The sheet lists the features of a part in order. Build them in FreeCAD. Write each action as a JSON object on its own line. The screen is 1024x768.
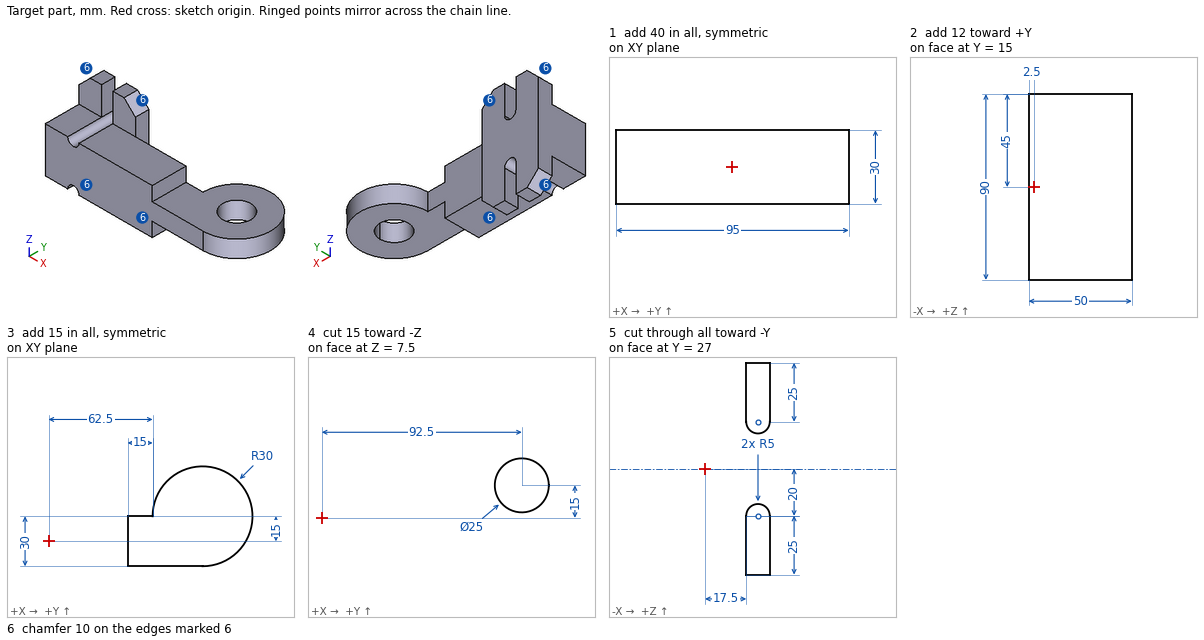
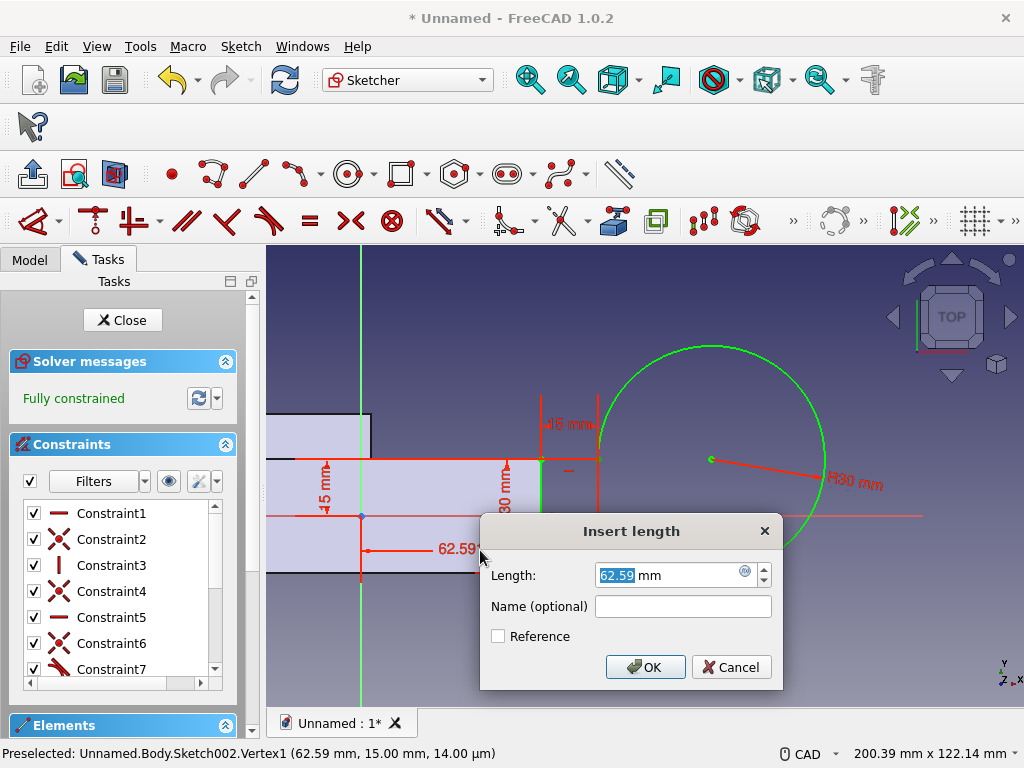
{"action": "type", "text": "62.5"}
{"action": "key", "text": "Return"}
{"action": "key", "text": "Escape"}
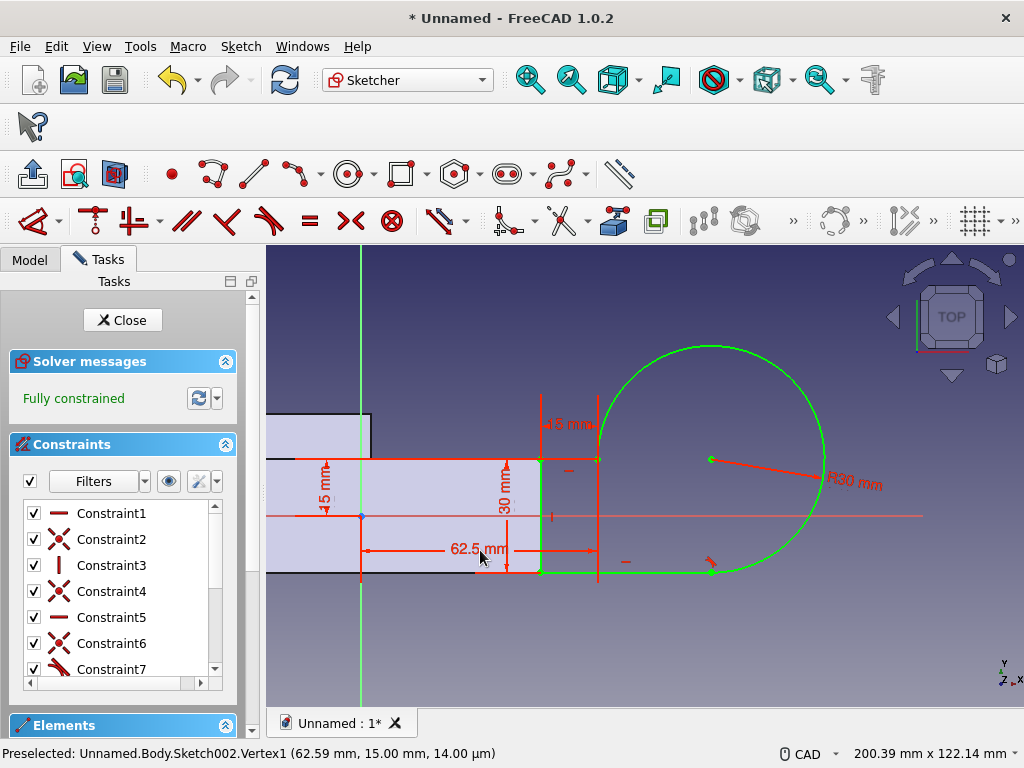
{"action": "left_click", "coordinate": [123, 320]}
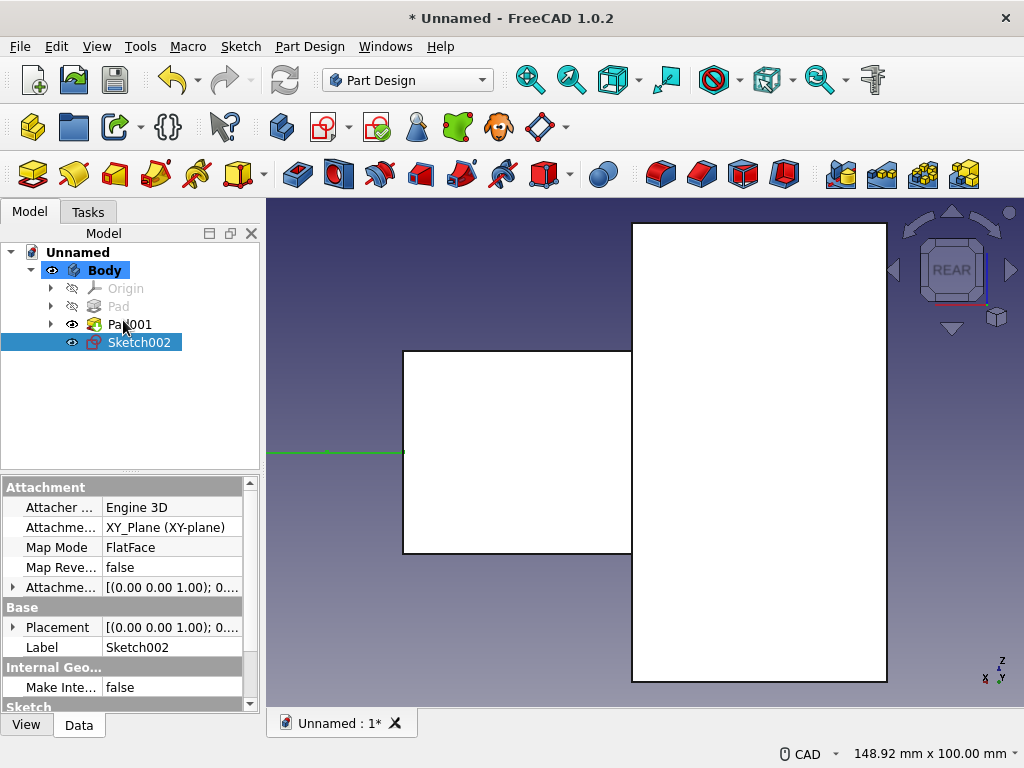
{"action": "left_click", "coordinate": [33, 174]}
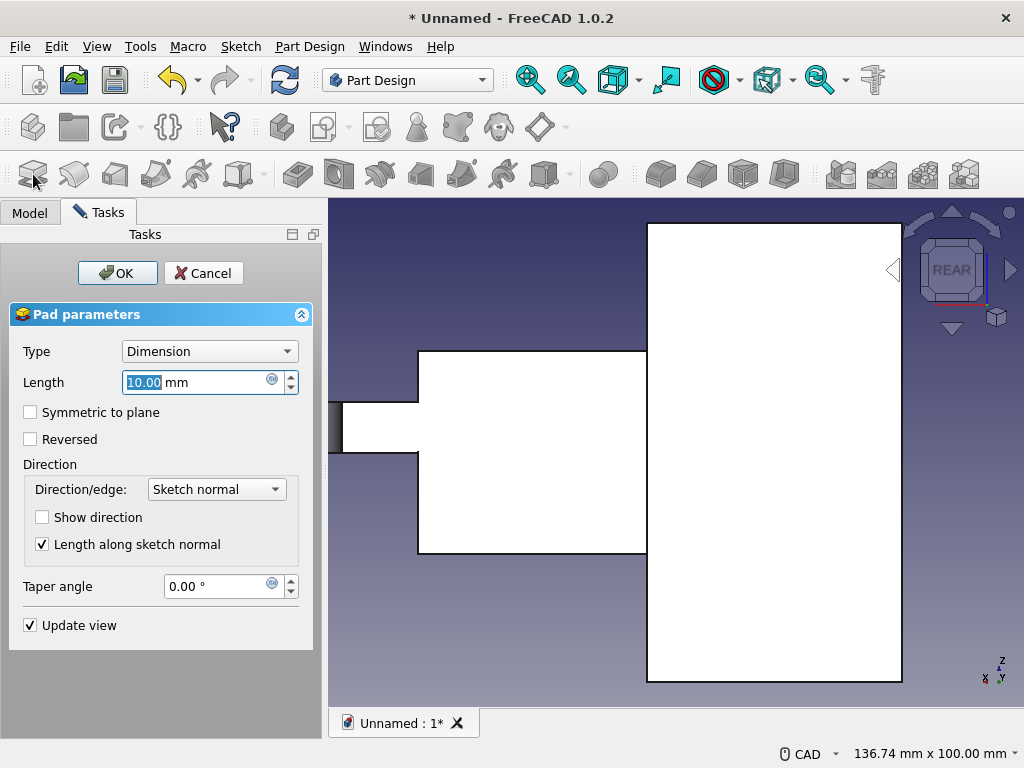
{"action": "type", "text": "15"}
{"action": "key", "text": "Tab"}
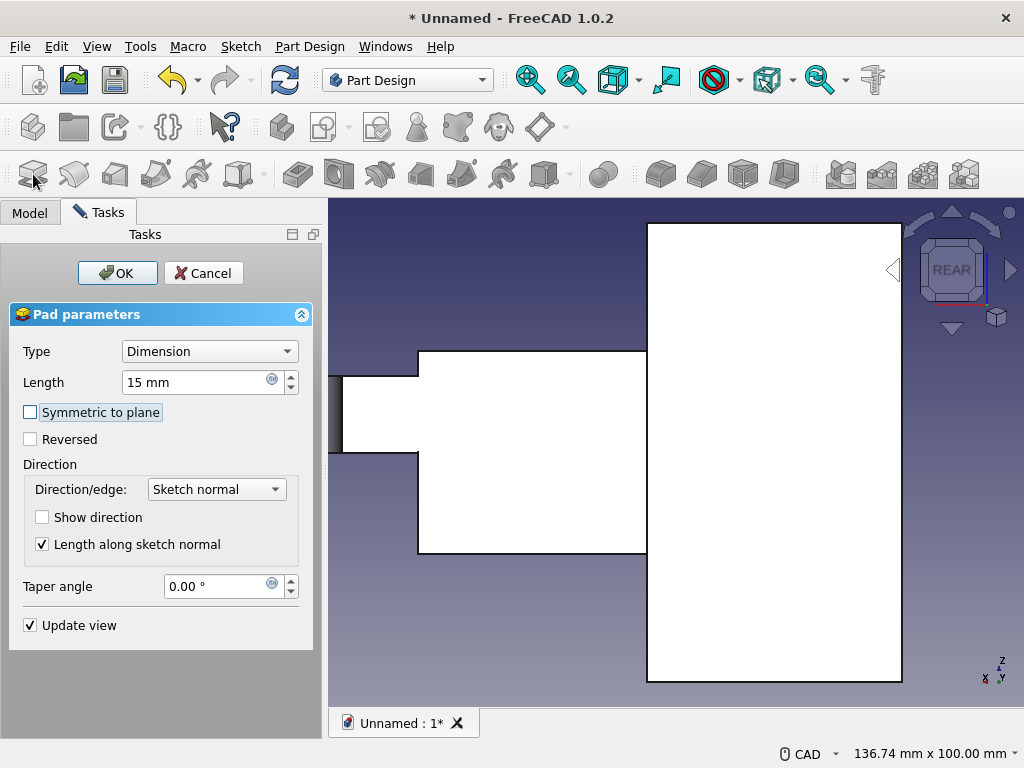
{"action": "left_click", "coordinate": [31, 412]}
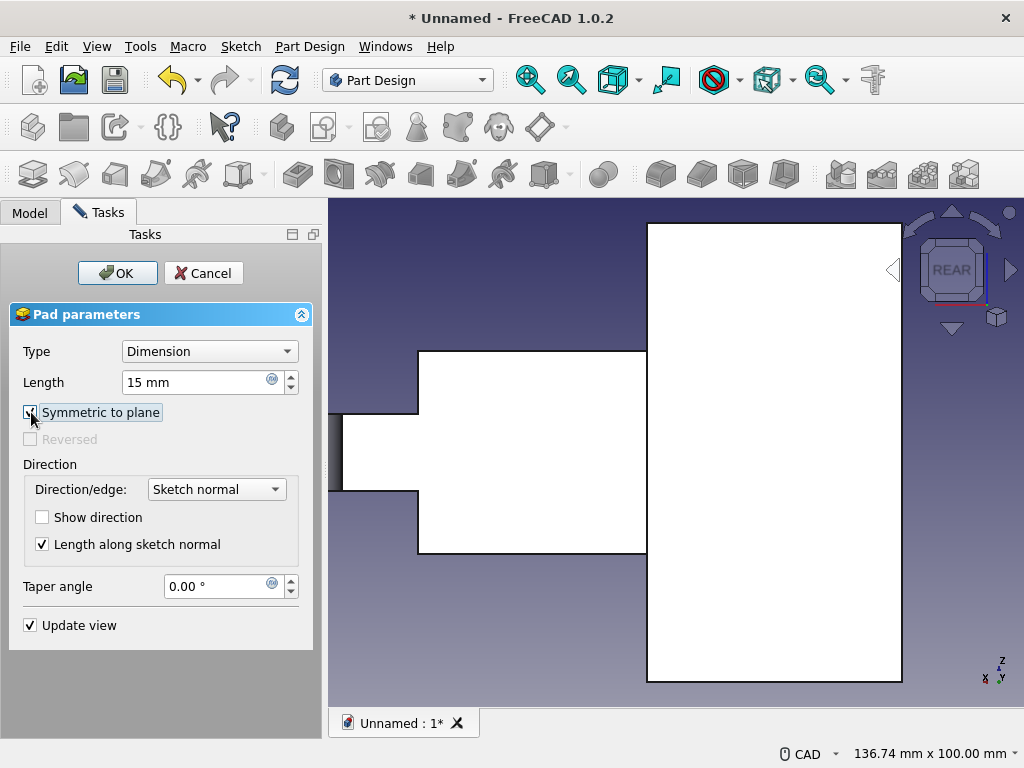
{"action": "left_click", "coordinate": [118, 273]}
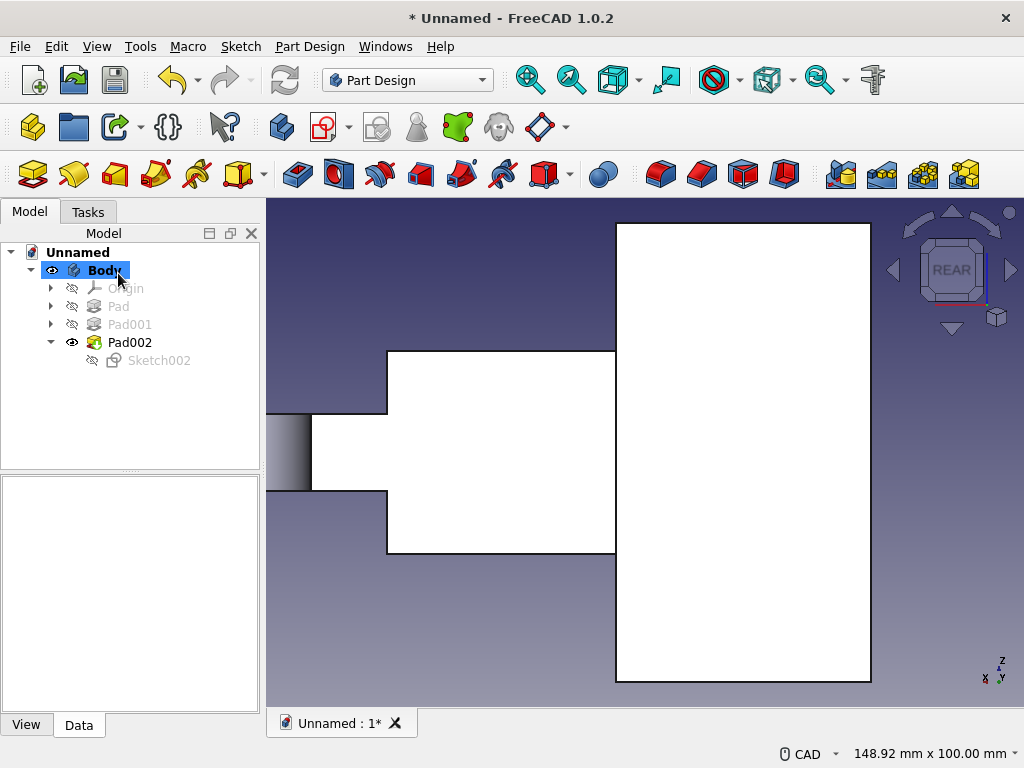
{"action": "left_click", "coordinate": [531, 80]}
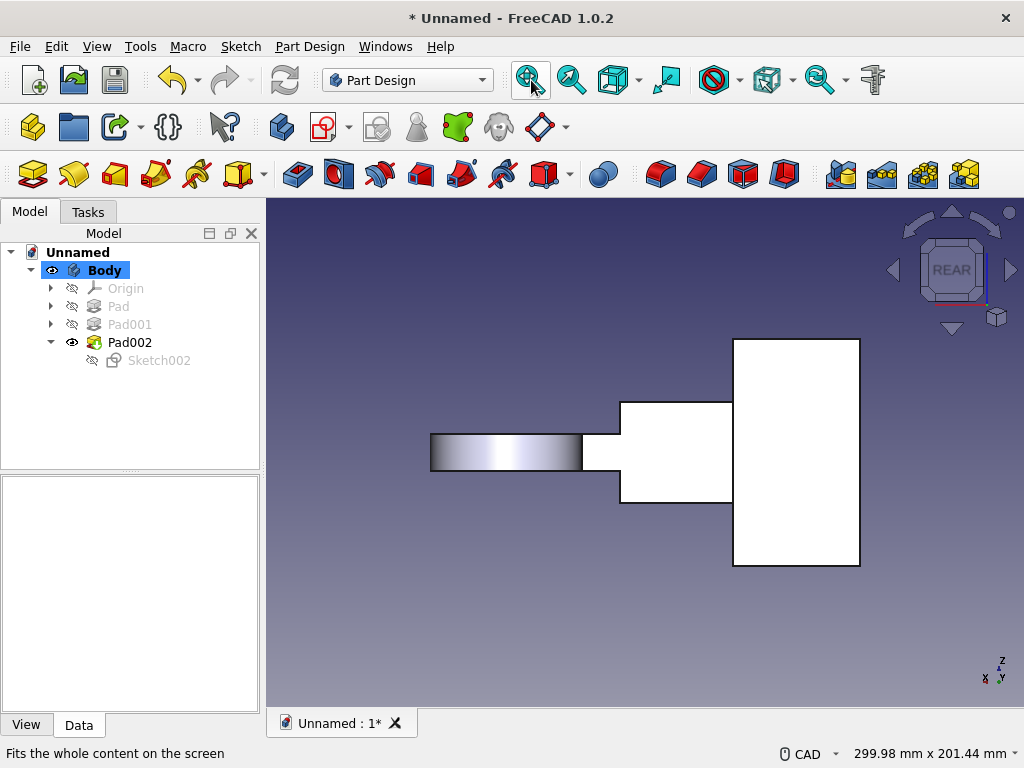
{"action": "key", "text": "0"}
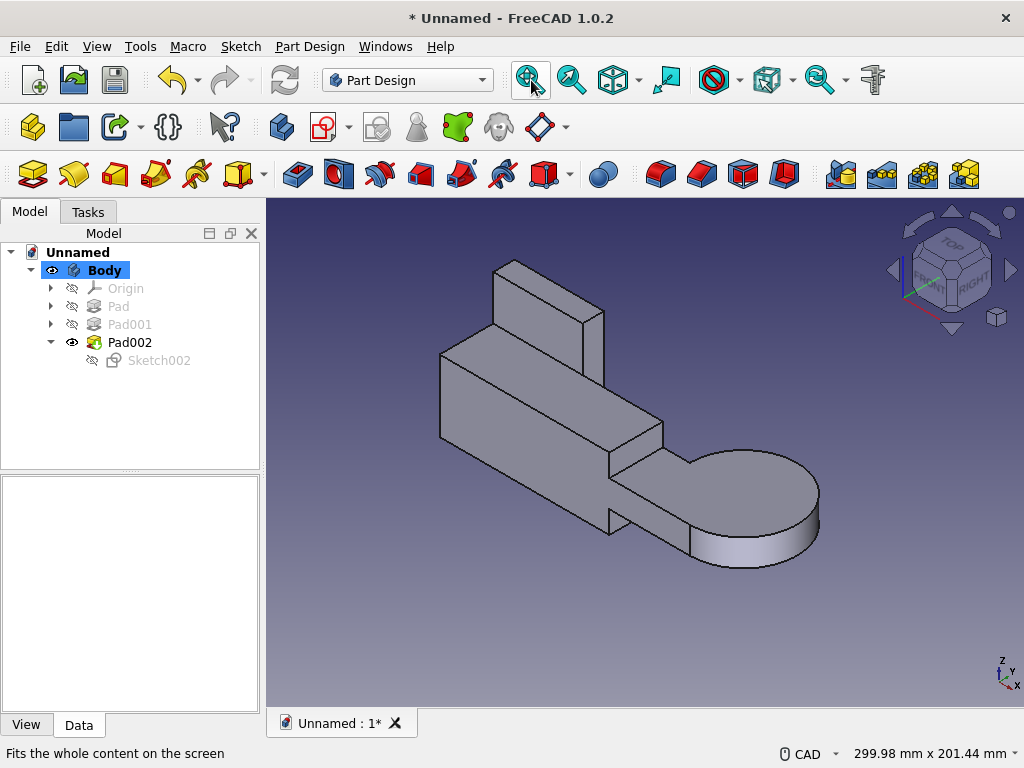
{"action": "left_click", "coordinate": [749, 496]}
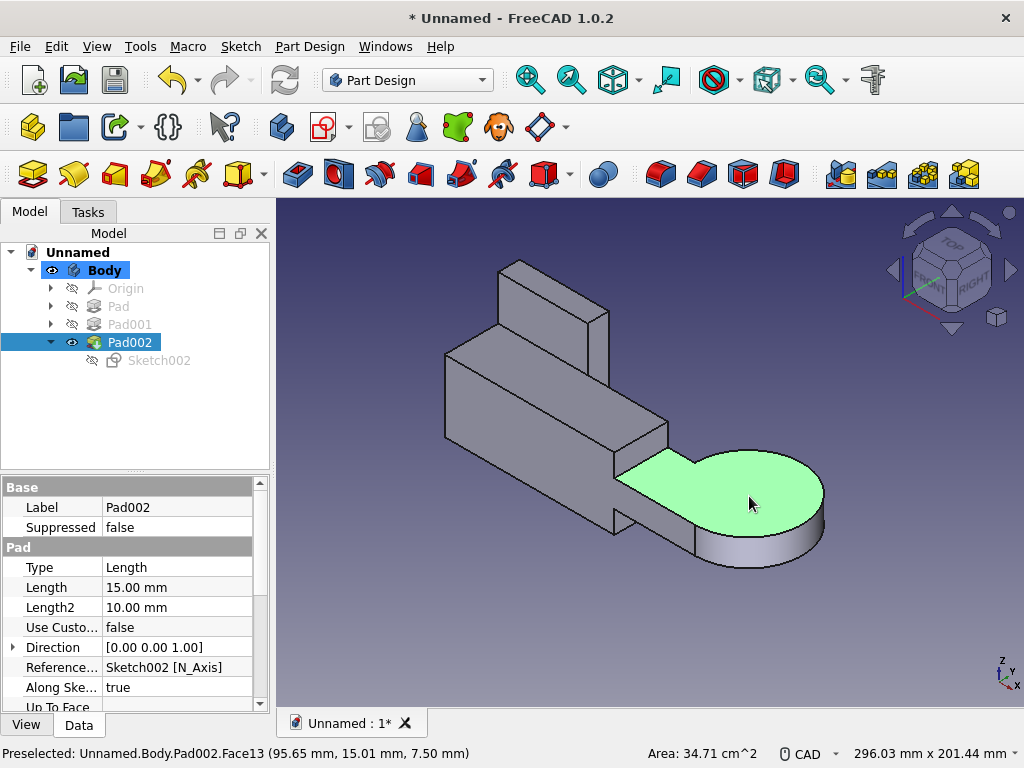
{"action": "left_click", "coordinate": [322, 128]}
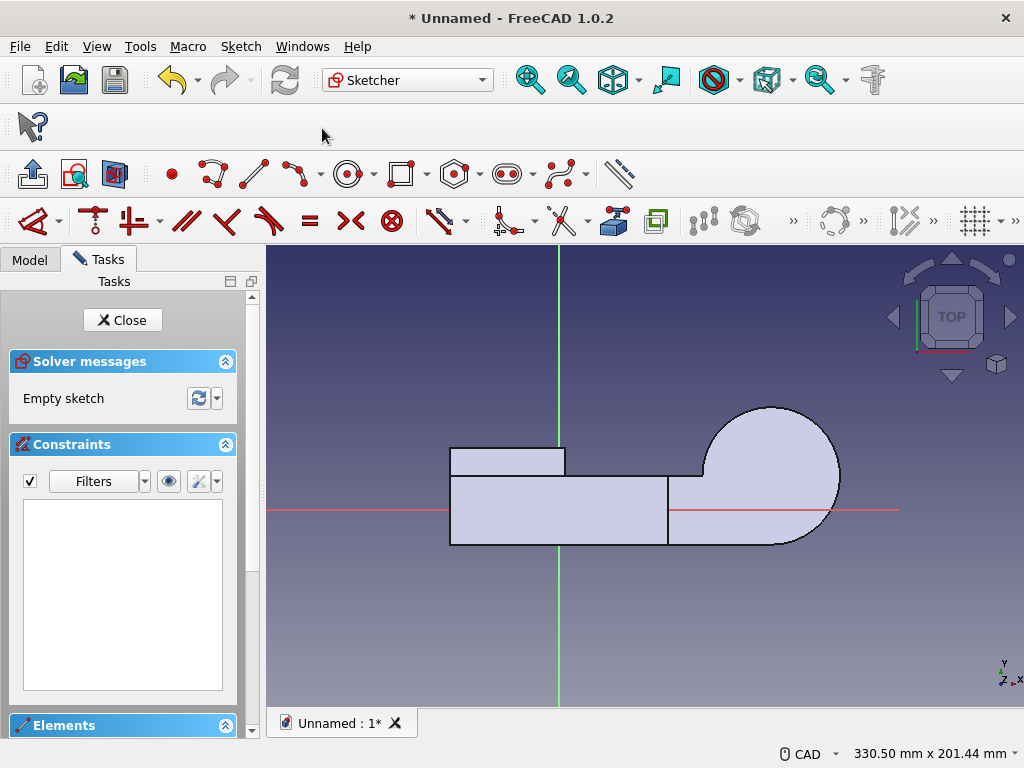
{"action": "left_click", "coordinate": [115, 174]}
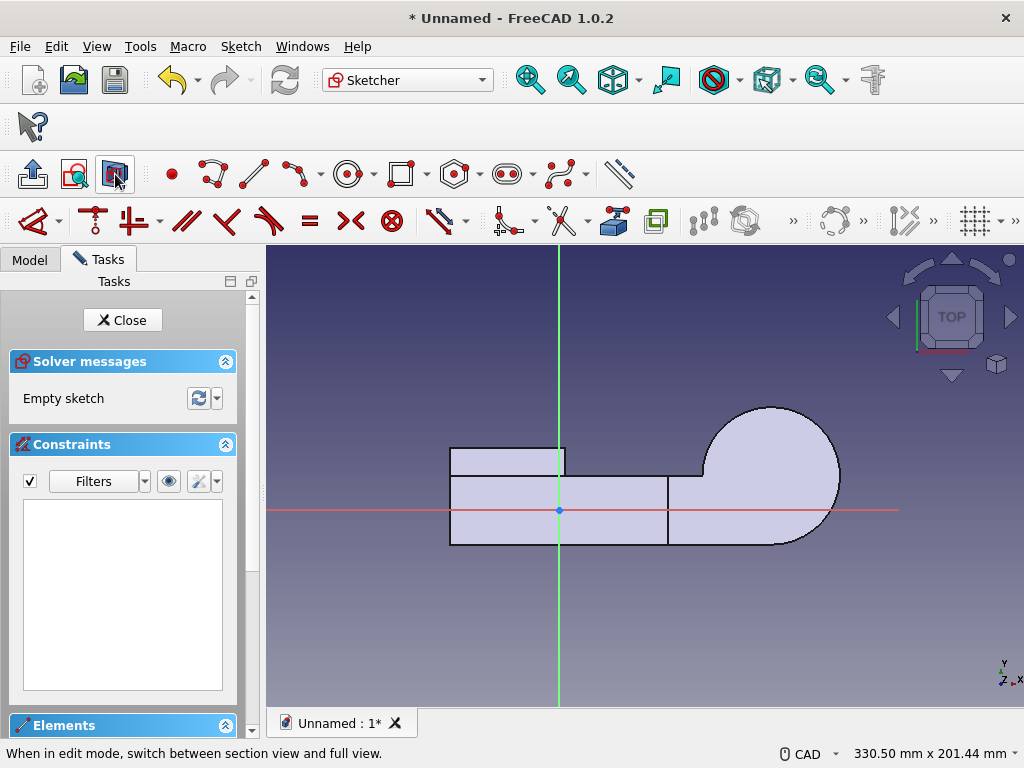
{"action": "scroll", "coordinate": [820, 476], "scroll_direction": "up", "scroll_amount": 8}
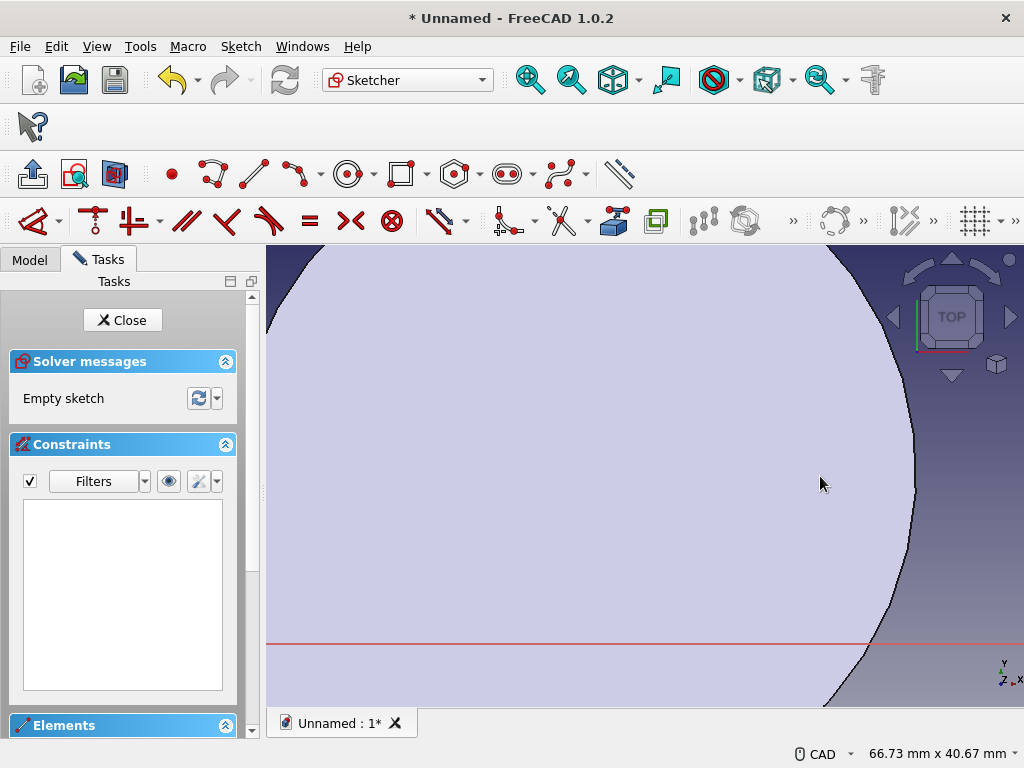
{"action": "left_click", "coordinate": [348, 174]}